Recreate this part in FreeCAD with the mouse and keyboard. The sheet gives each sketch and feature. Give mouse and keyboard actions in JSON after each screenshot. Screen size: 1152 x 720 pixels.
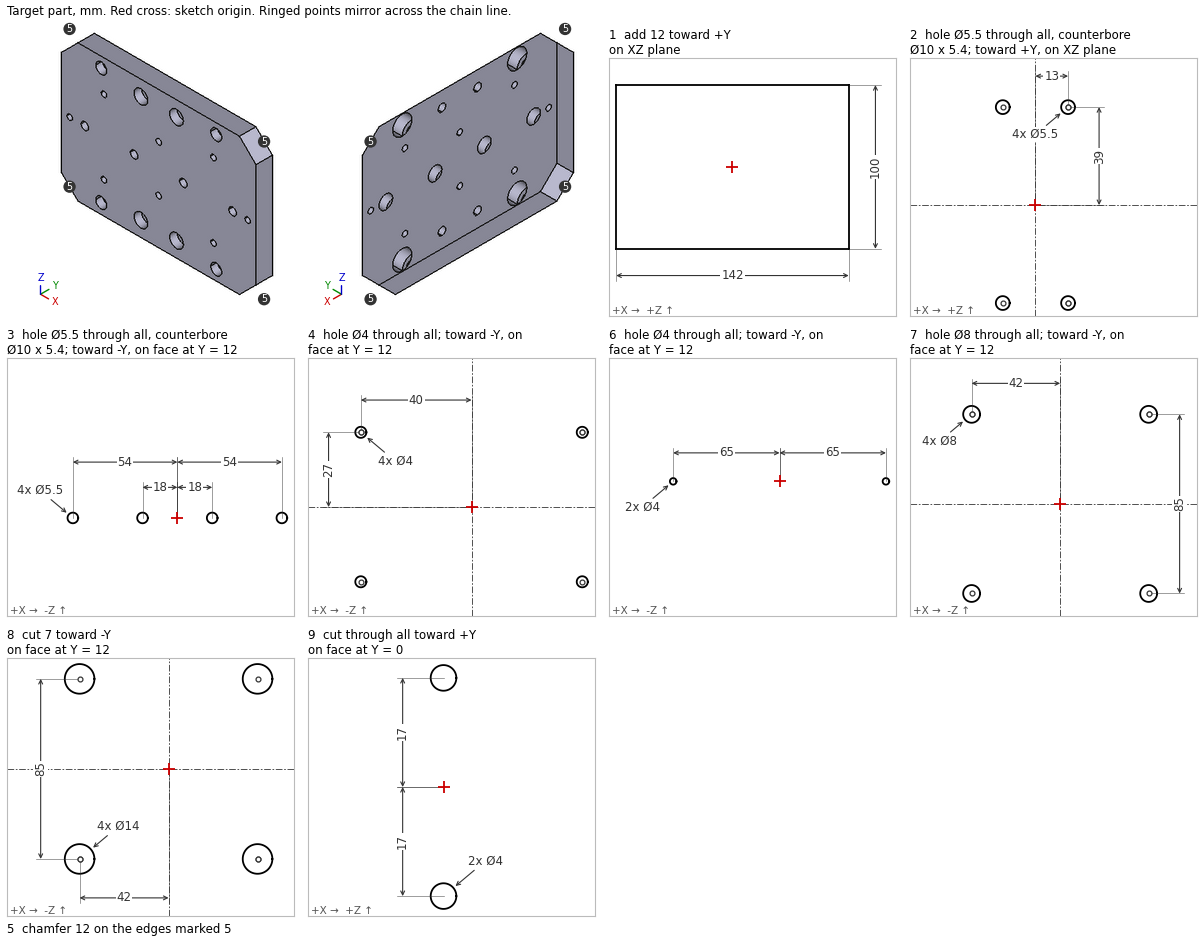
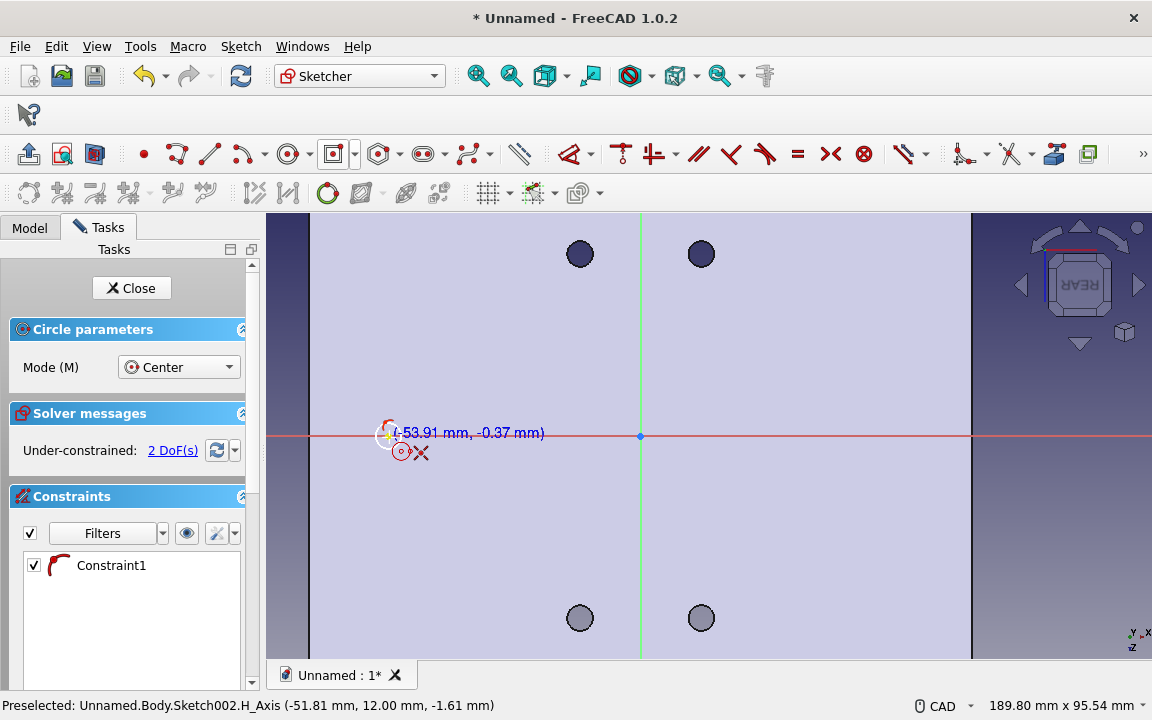
{"action": "scroll", "coordinate": [893, 436], "scroll_direction": "up", "scroll_amount": 3}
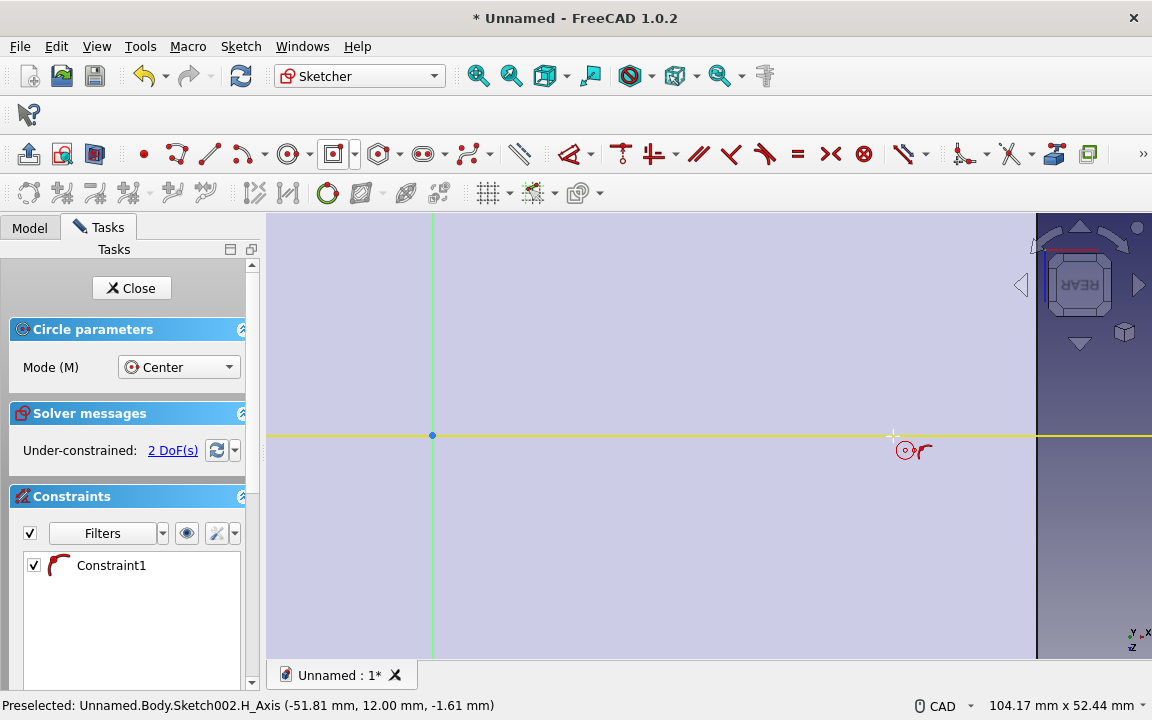
{"action": "left_click", "coordinate": [892, 436]}
{"action": "left_click", "coordinate": [909, 419]}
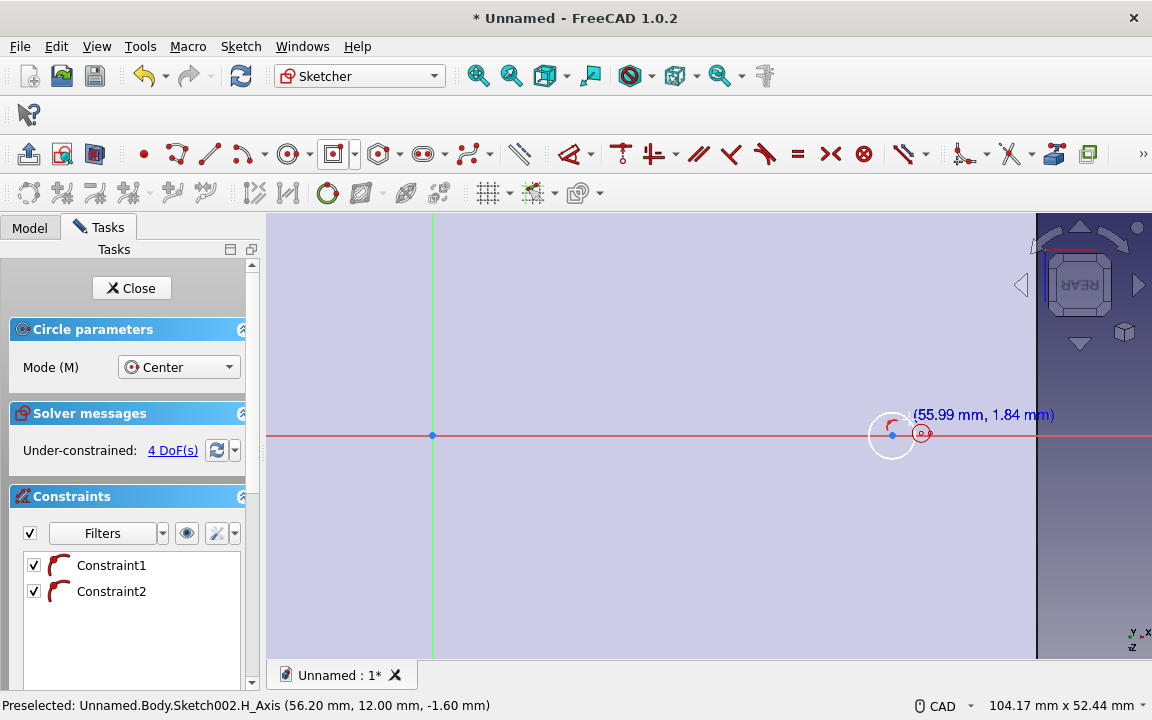
{"action": "scroll", "coordinate": [893, 436], "scroll_direction": "down", "scroll_amount": 3}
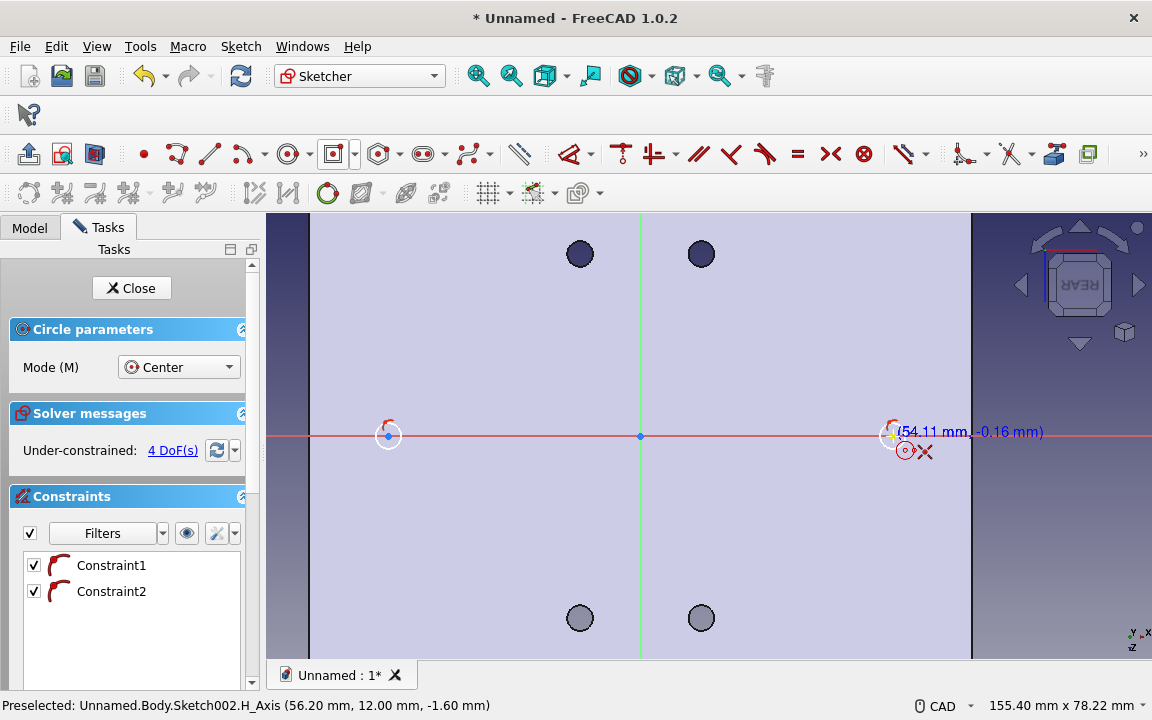
{"action": "scroll", "coordinate": [557, 436], "scroll_direction": "up", "scroll_amount": 3}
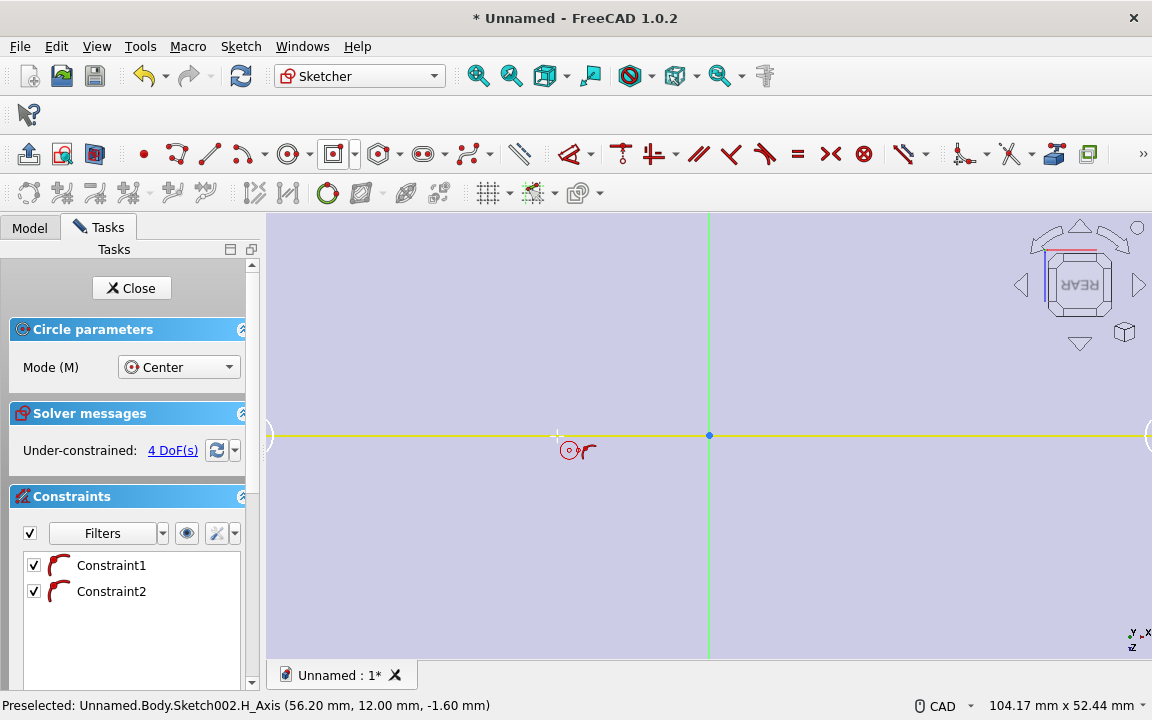
{"action": "left_click", "coordinate": [556, 436]}
{"action": "left_click", "coordinate": [573, 419]}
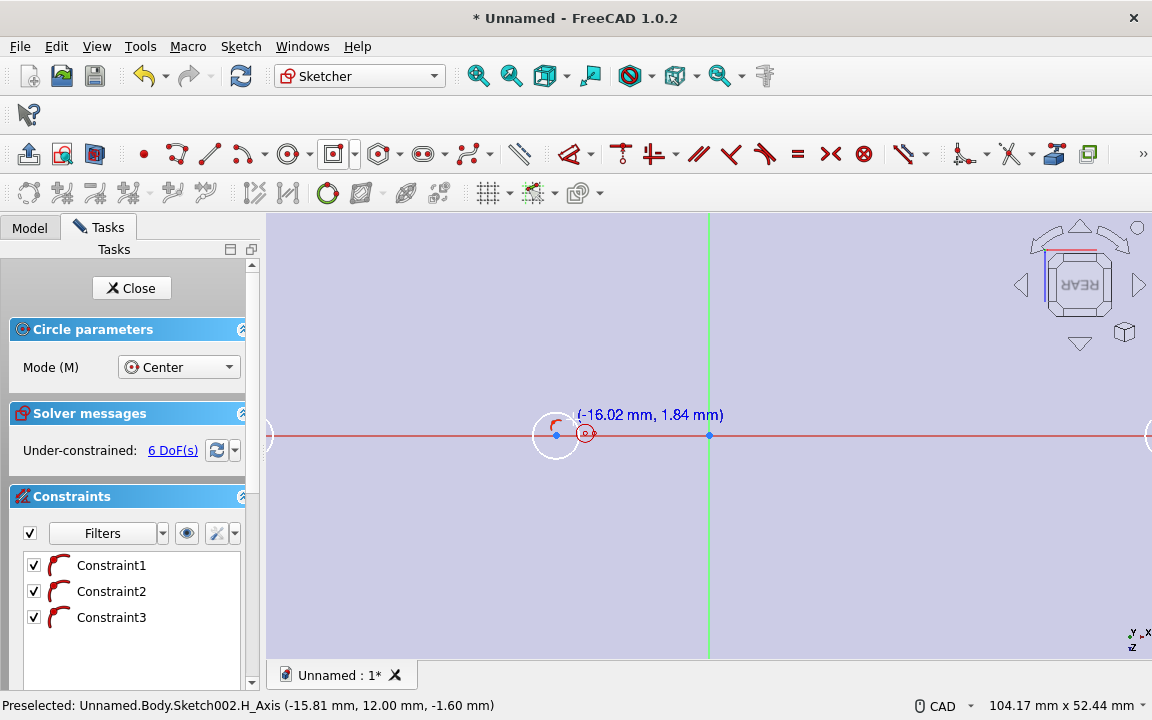
{"action": "left_click", "coordinate": [862, 436]}
{"action": "left_click", "coordinate": [879, 419]}
{"action": "key", "text": "Escape"}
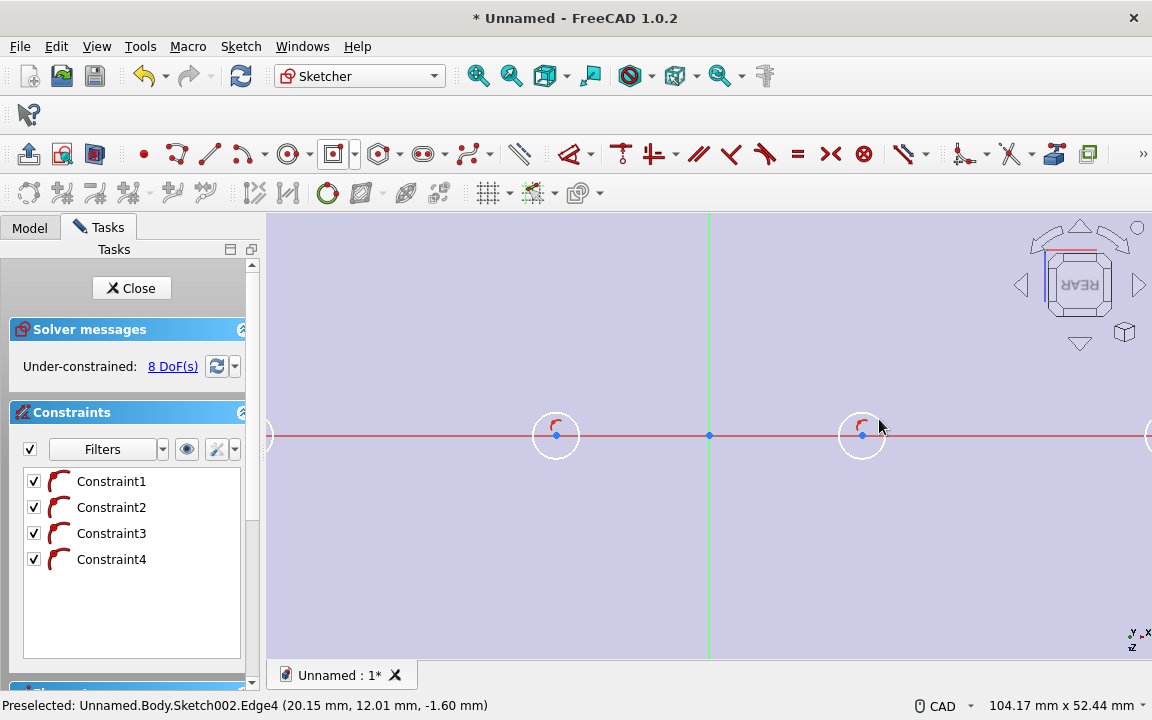
{"action": "scroll", "coordinate": [557, 436], "scroll_direction": "down", "scroll_amount": 3}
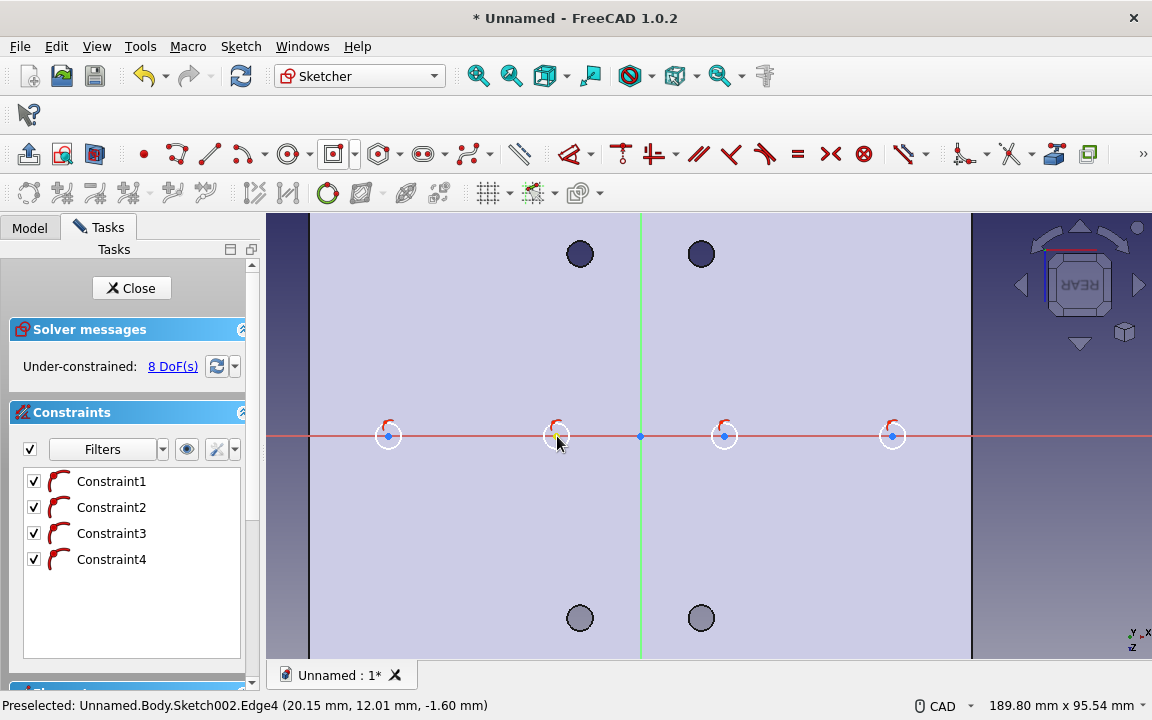
{"action": "scroll", "coordinate": [398, 427], "scroll_direction": "up", "scroll_amount": 3}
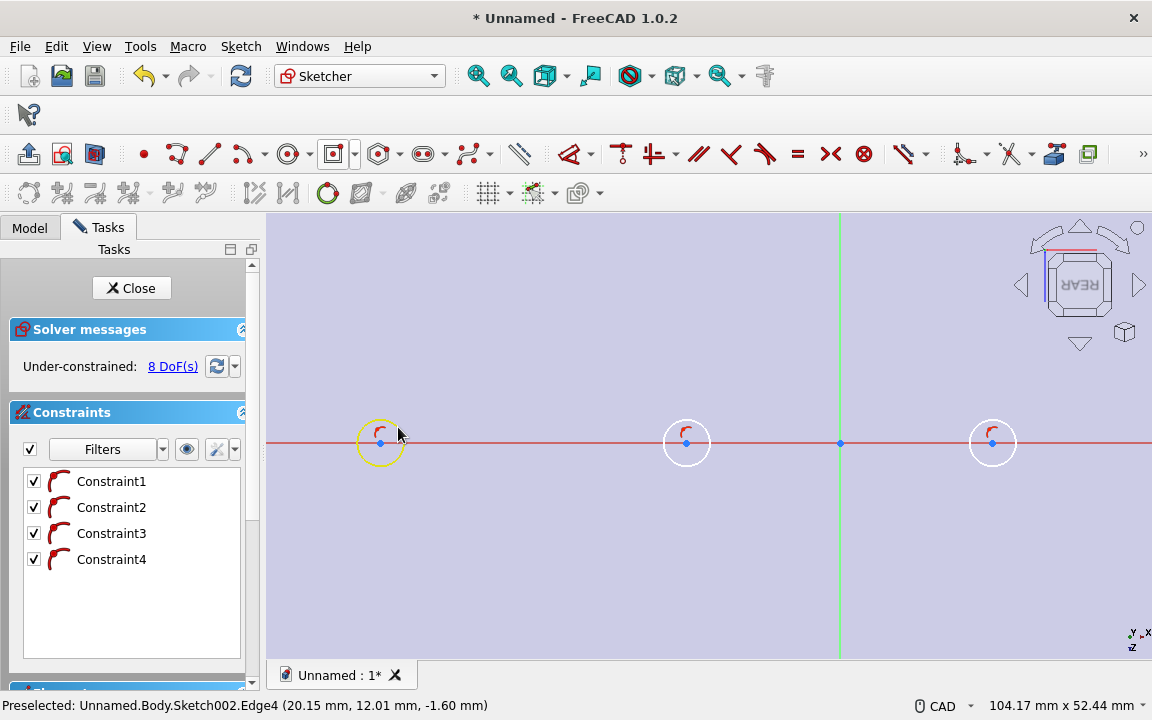
{"action": "left_click", "coordinate": [397, 427]}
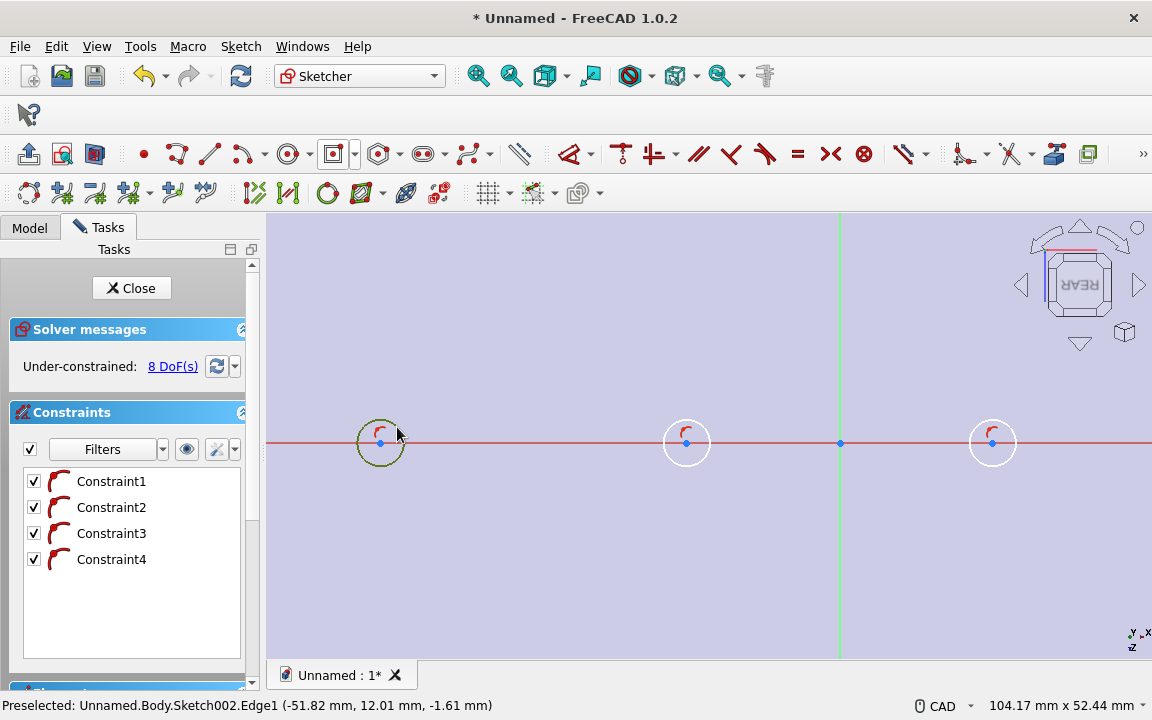
{"action": "scroll", "coordinate": [398, 427], "scroll_direction": "down", "scroll_amount": 3}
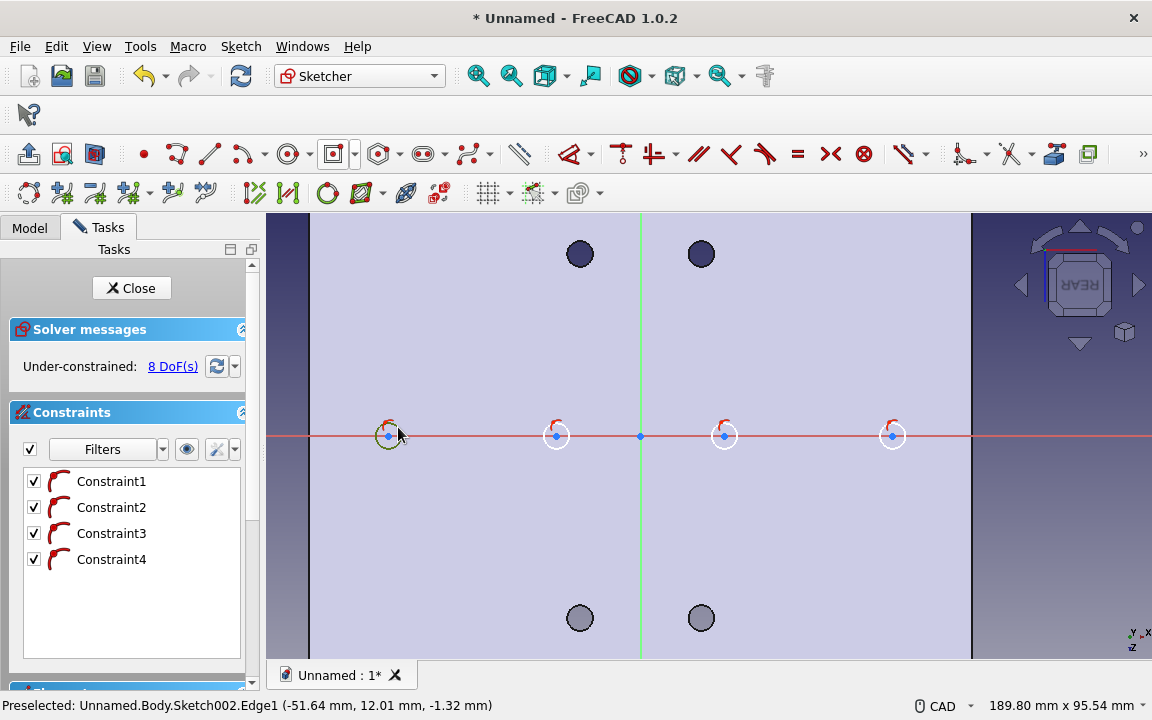
{"action": "scroll", "coordinate": [902, 427], "scroll_direction": "up", "scroll_amount": 3}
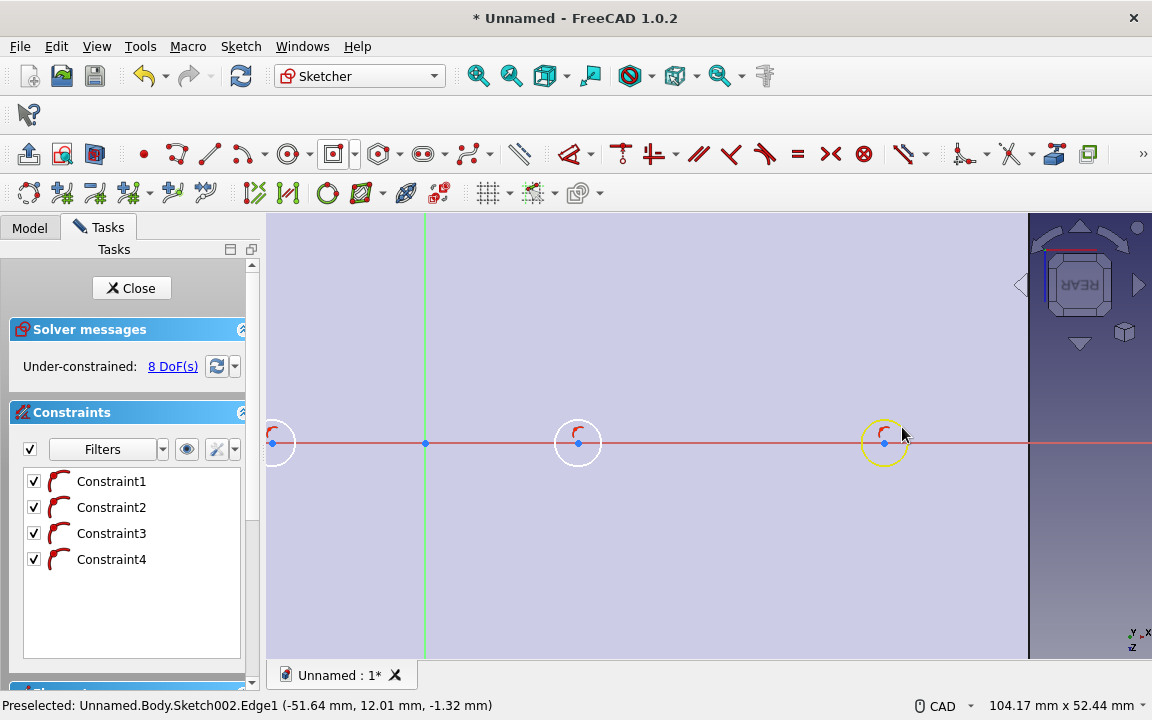
{"action": "left_click", "coordinate": [901, 427]}